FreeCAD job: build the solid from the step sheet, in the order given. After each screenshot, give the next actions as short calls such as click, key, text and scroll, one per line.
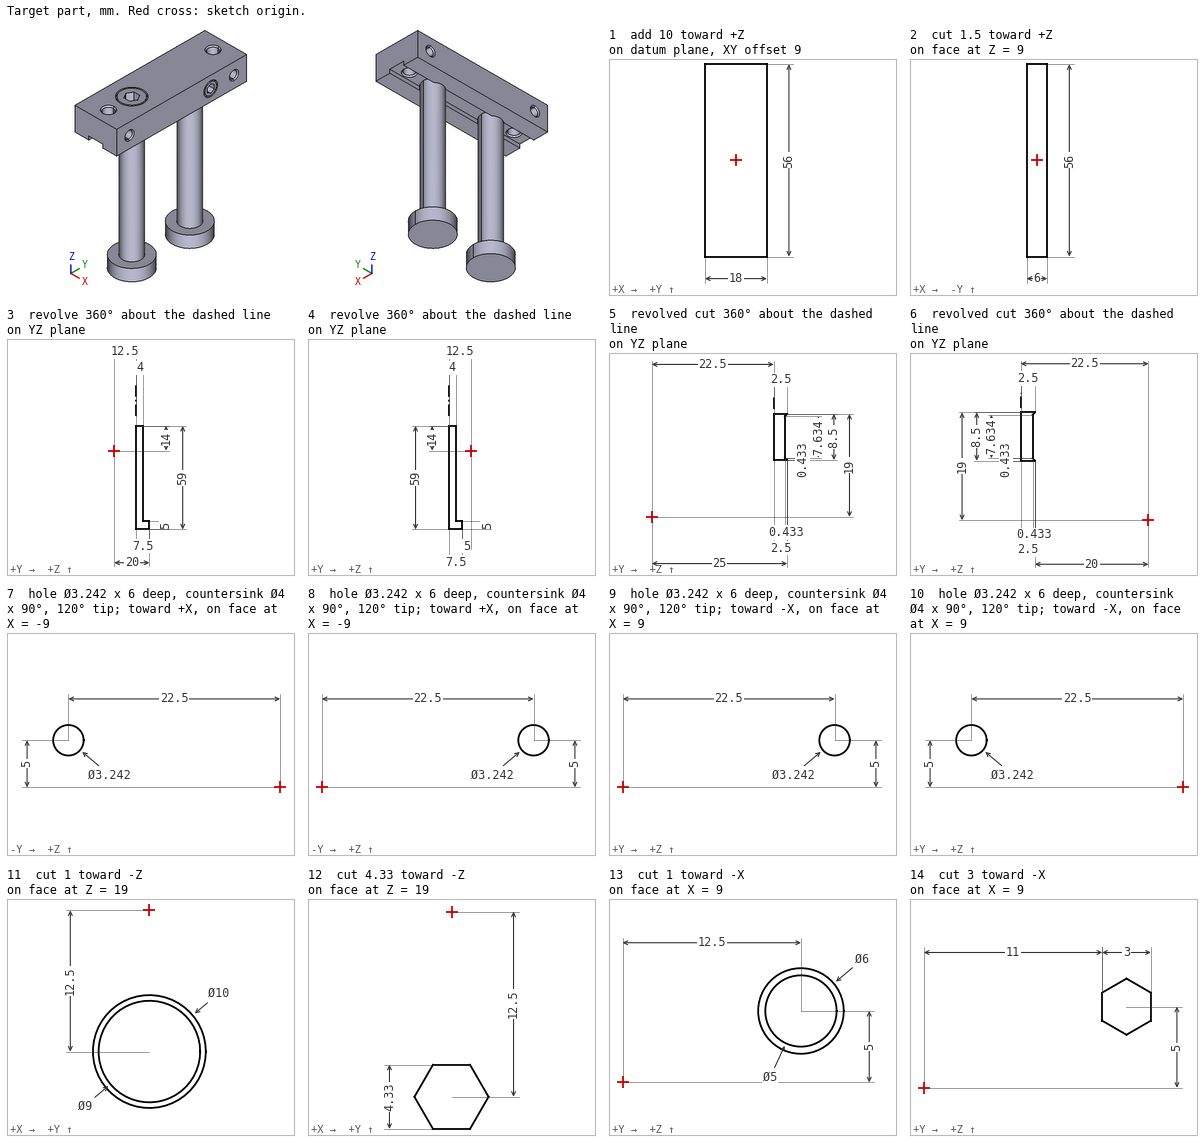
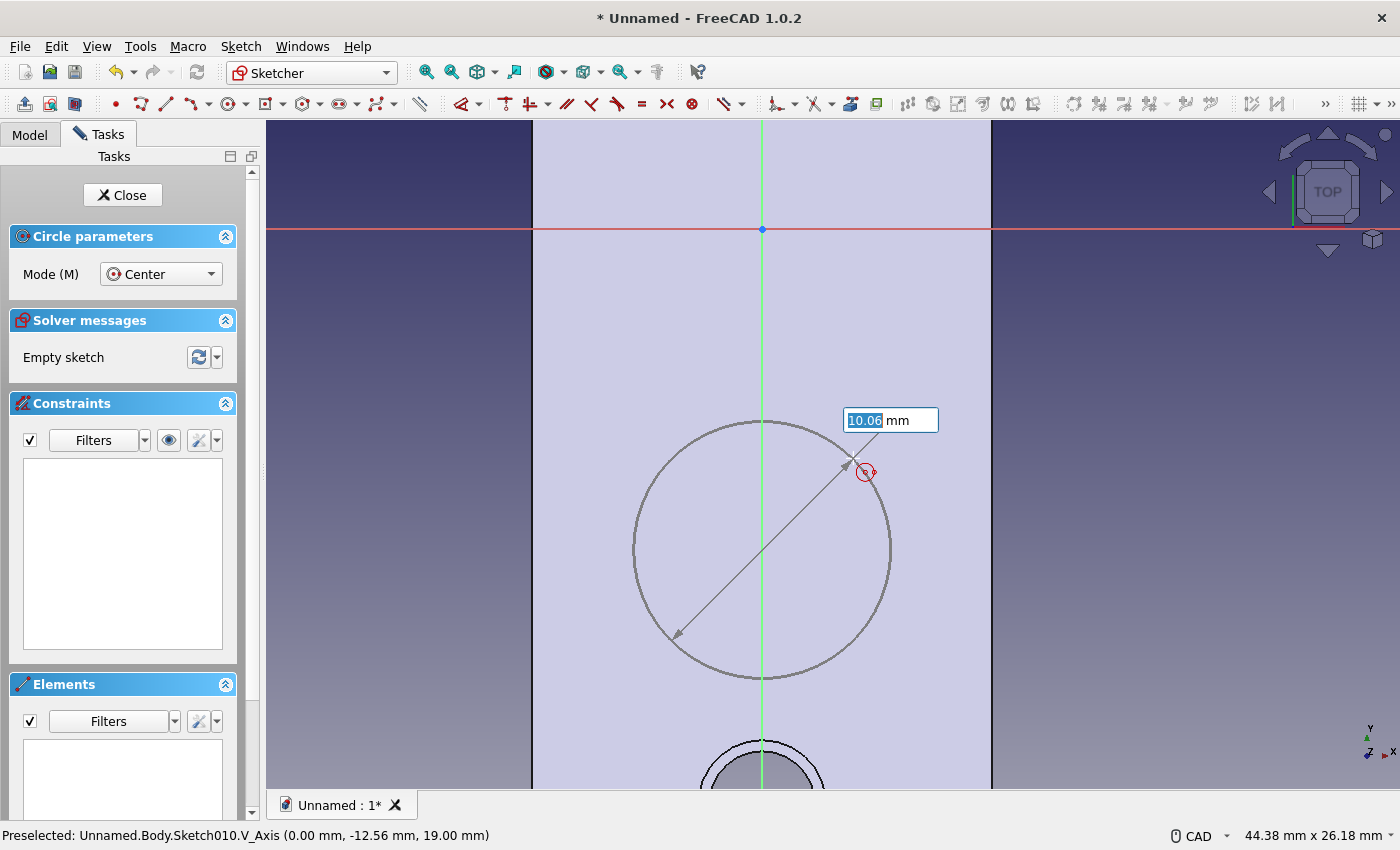
text(10)
key(Return)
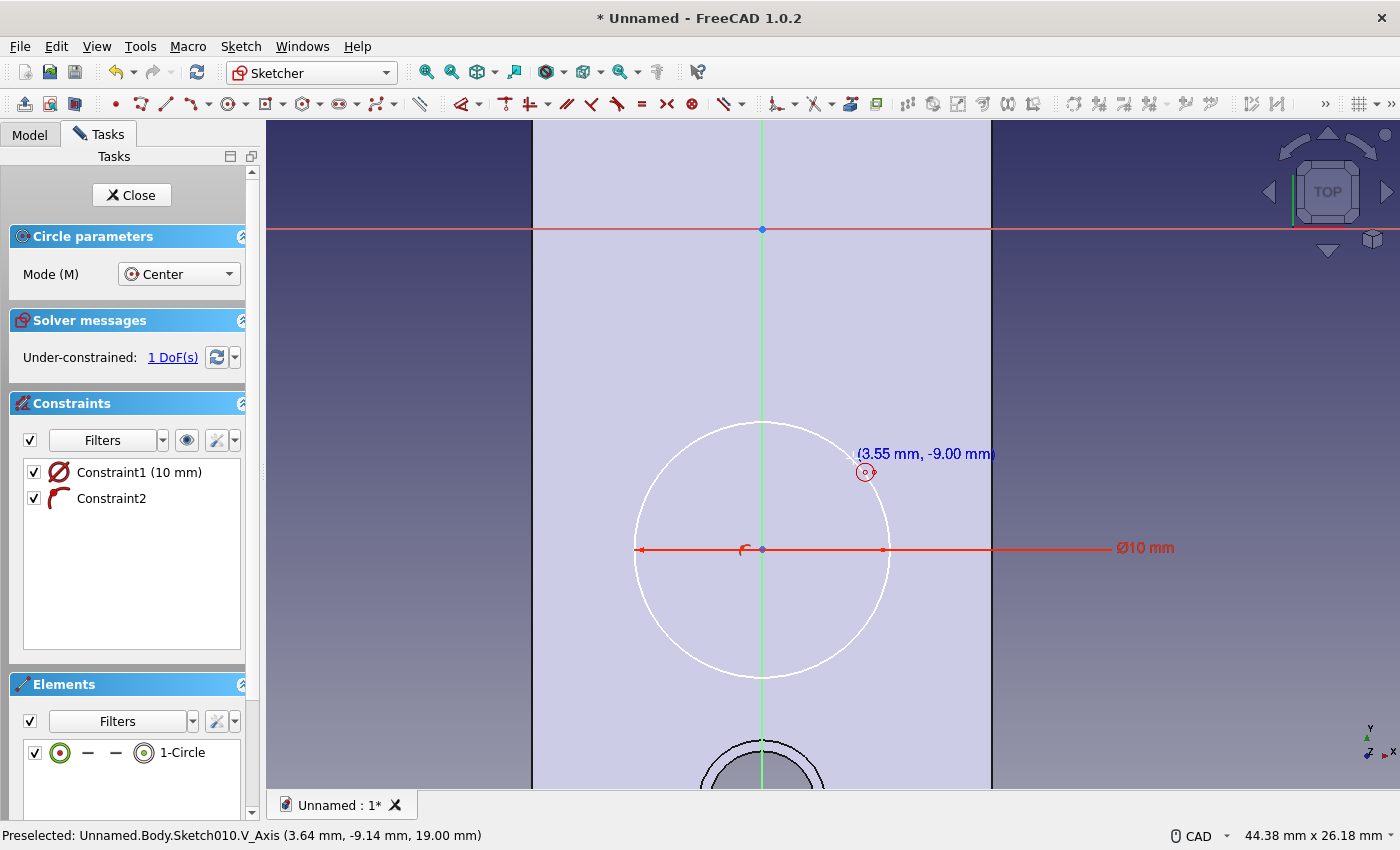
click(762, 550)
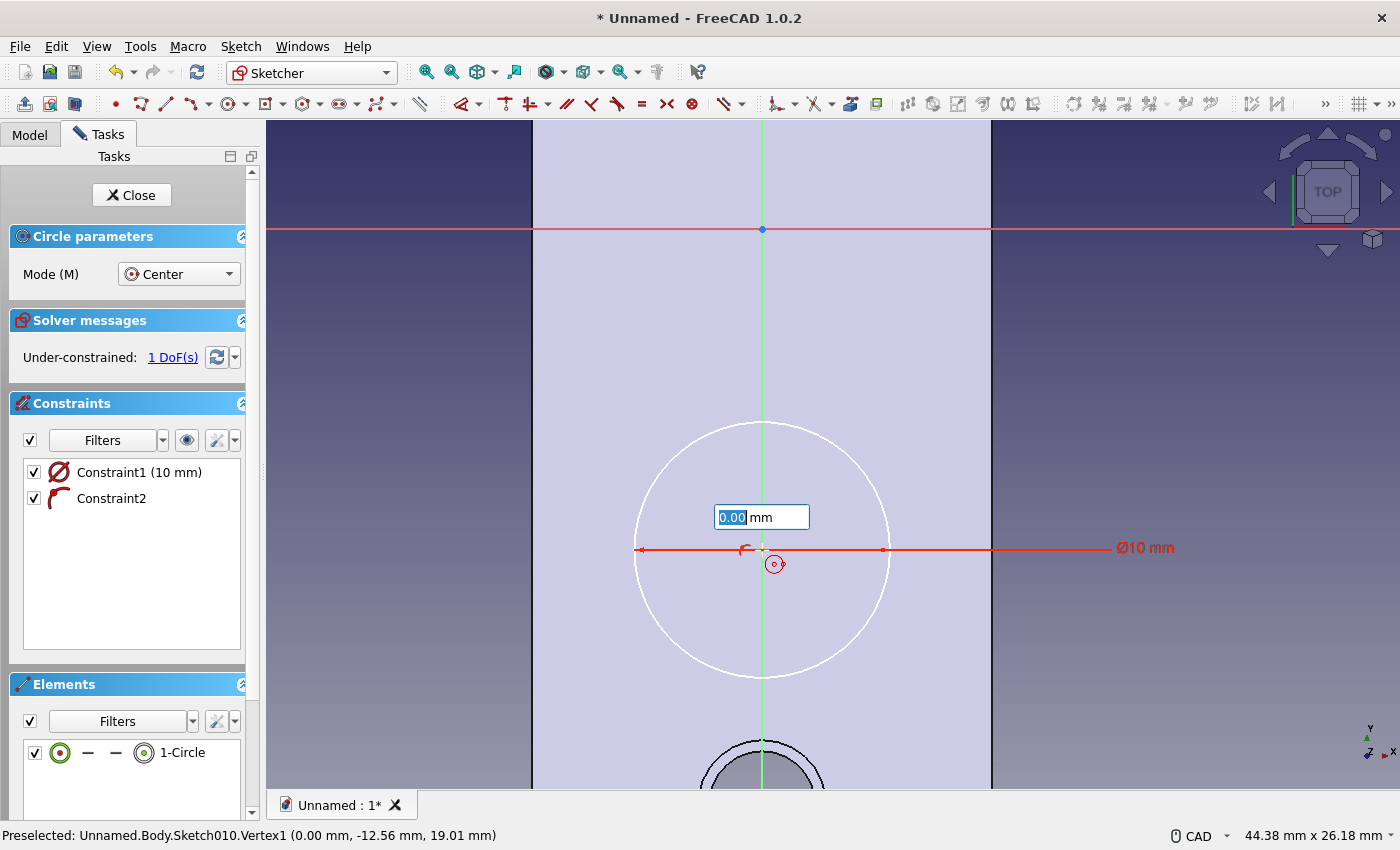
scroll(843, 630, up, 2)
move(843, 629)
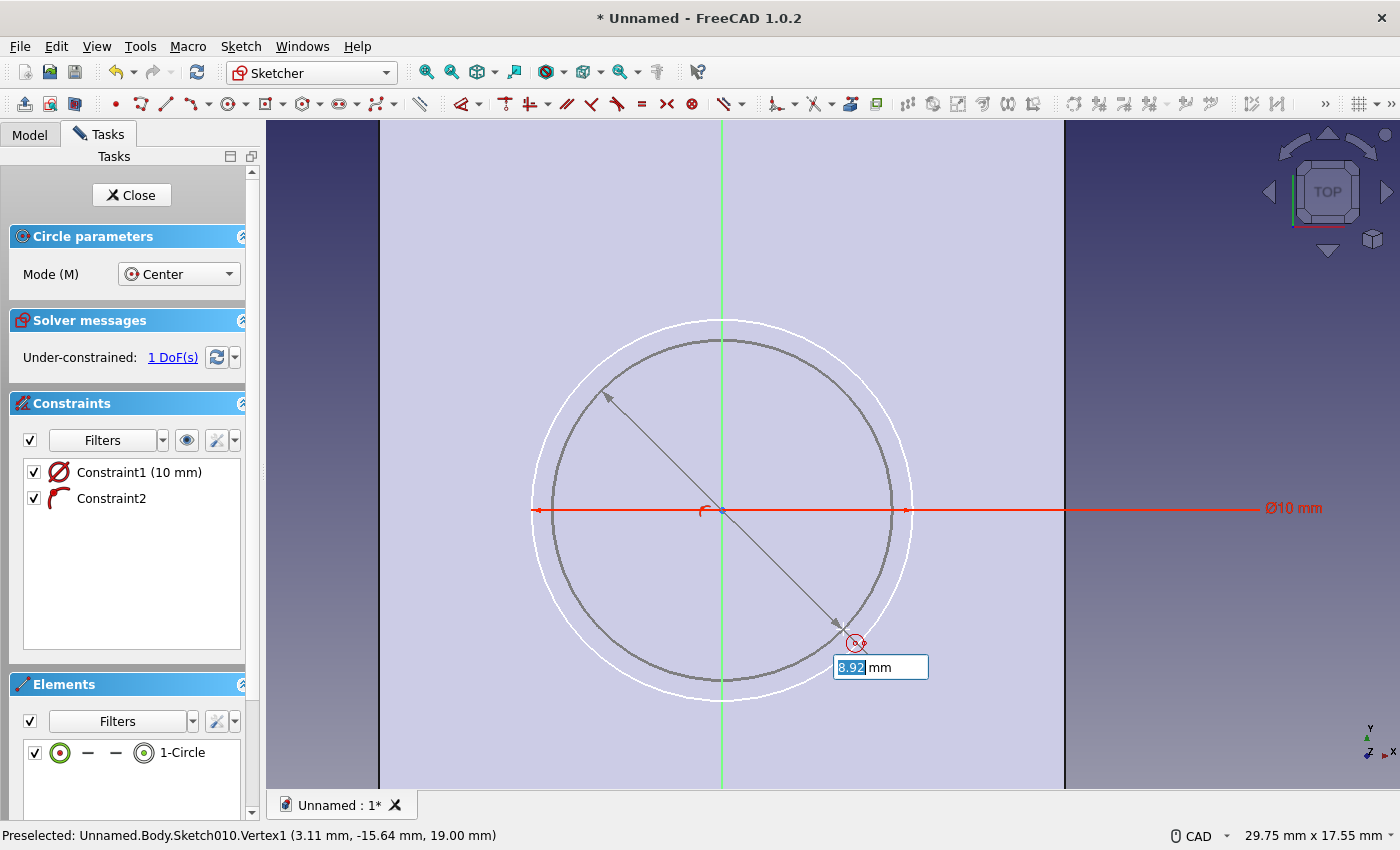
text(9)
key(Return)
key(Escape)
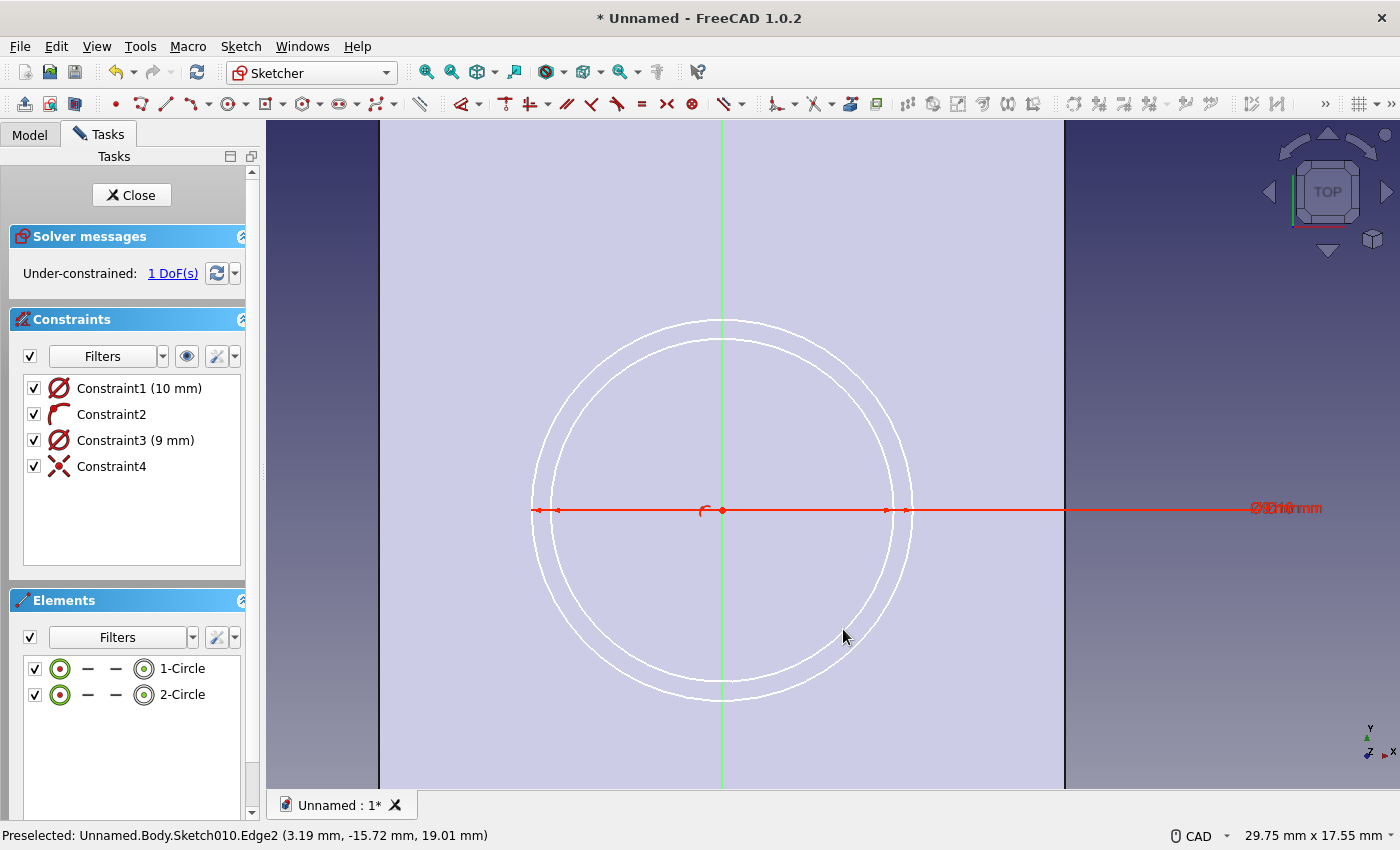
click(460, 104)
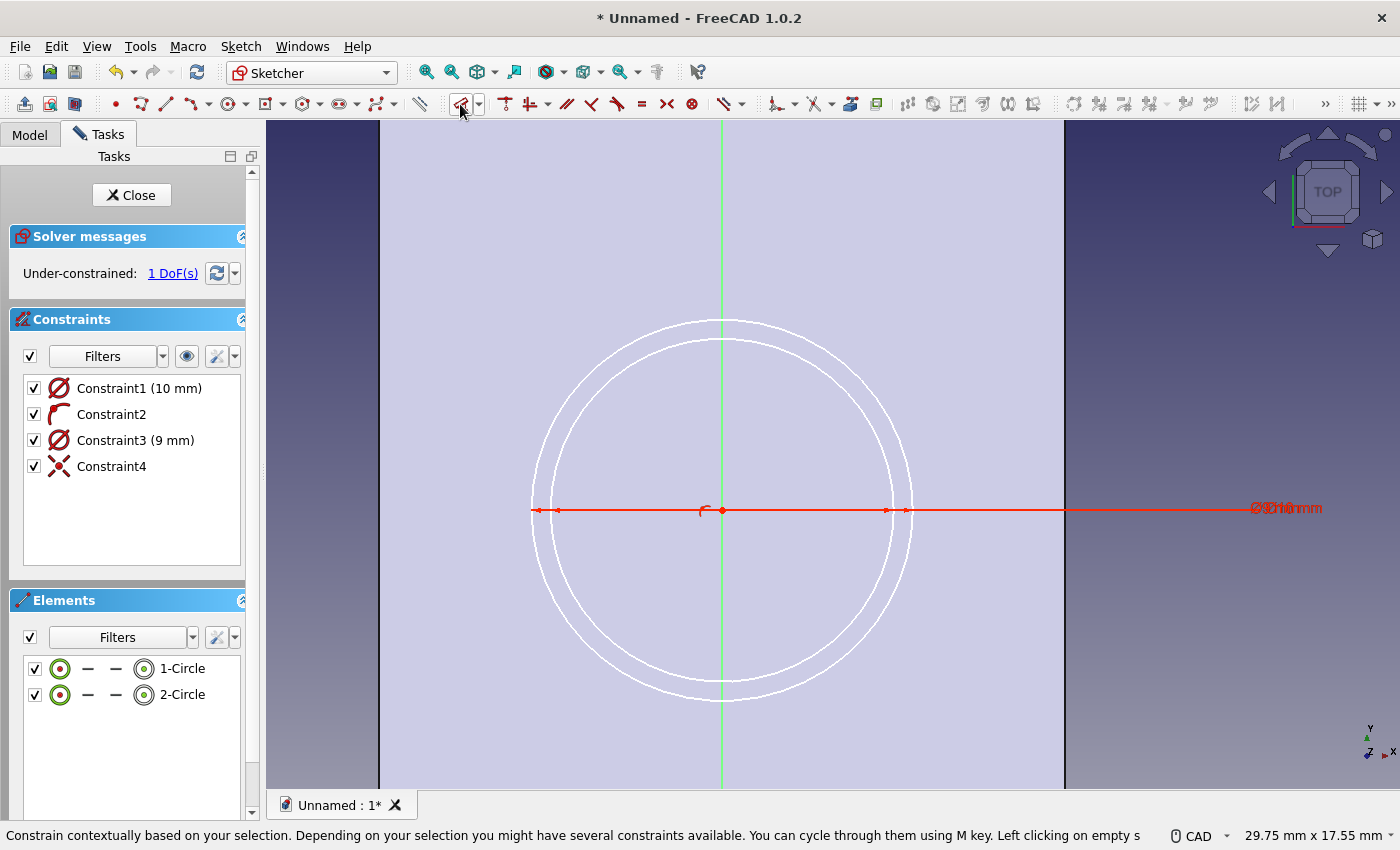
click(722, 510)
click(756, 246)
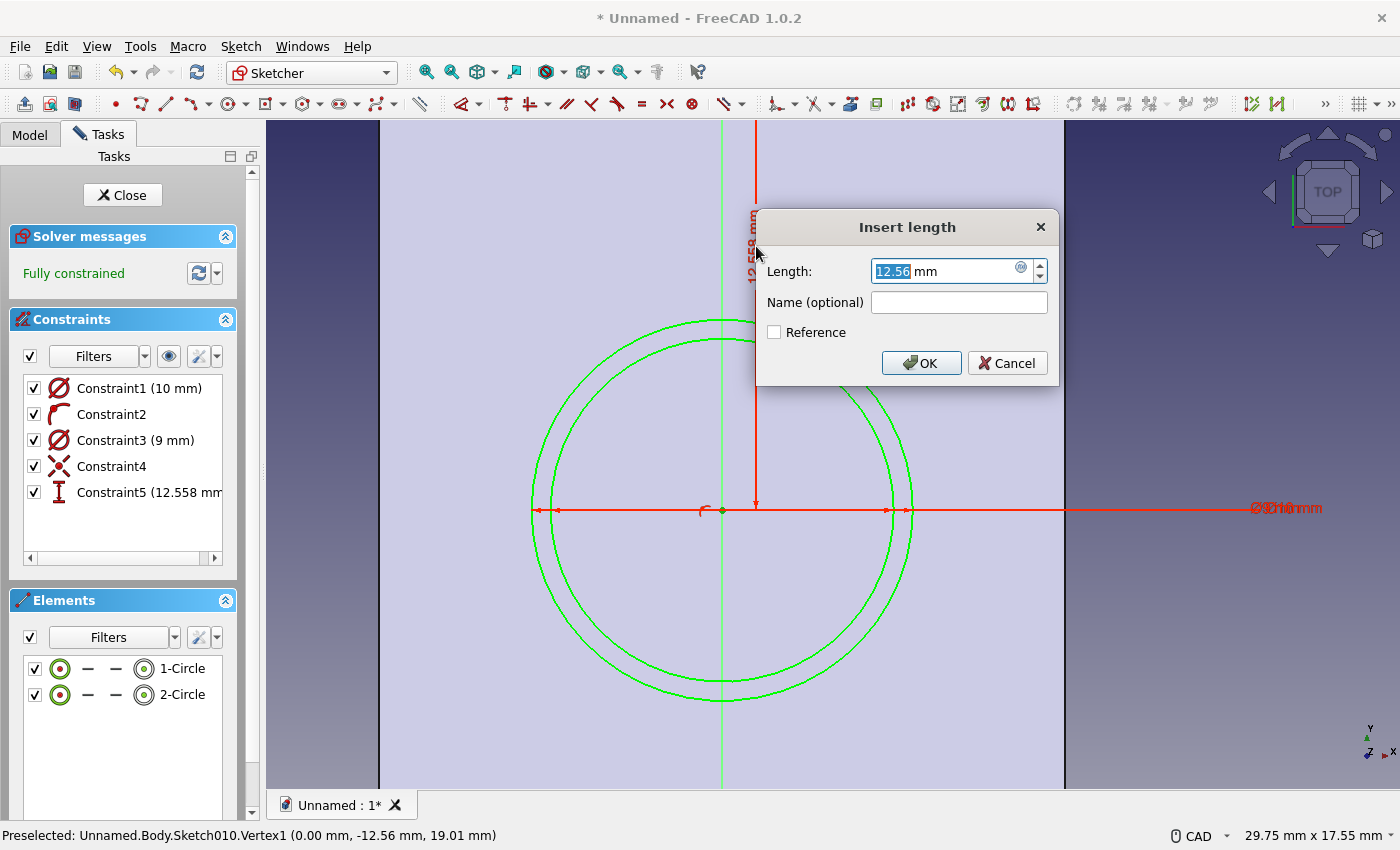
text(12.5)
key(Return)
key(Escape)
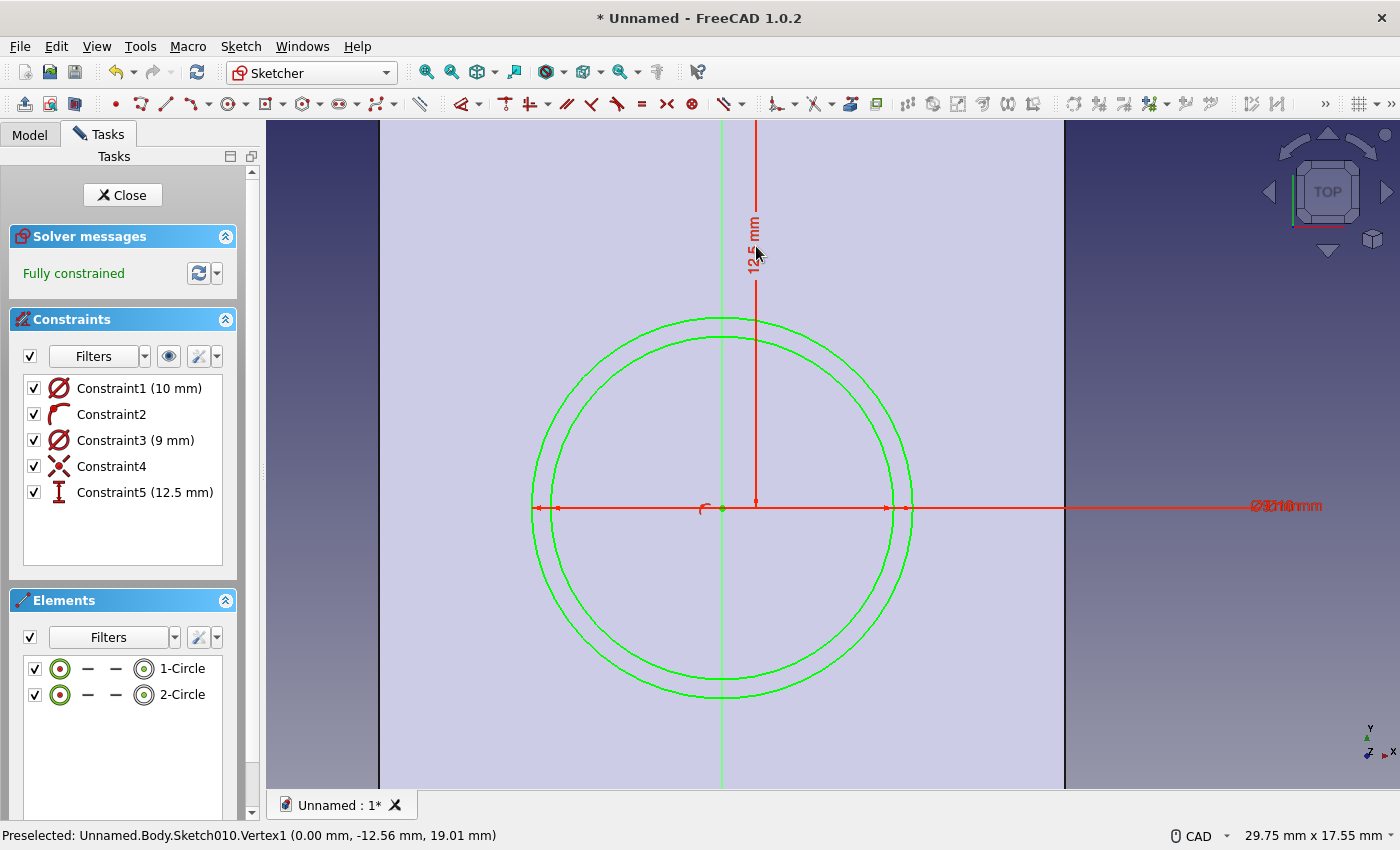
click(123, 195)